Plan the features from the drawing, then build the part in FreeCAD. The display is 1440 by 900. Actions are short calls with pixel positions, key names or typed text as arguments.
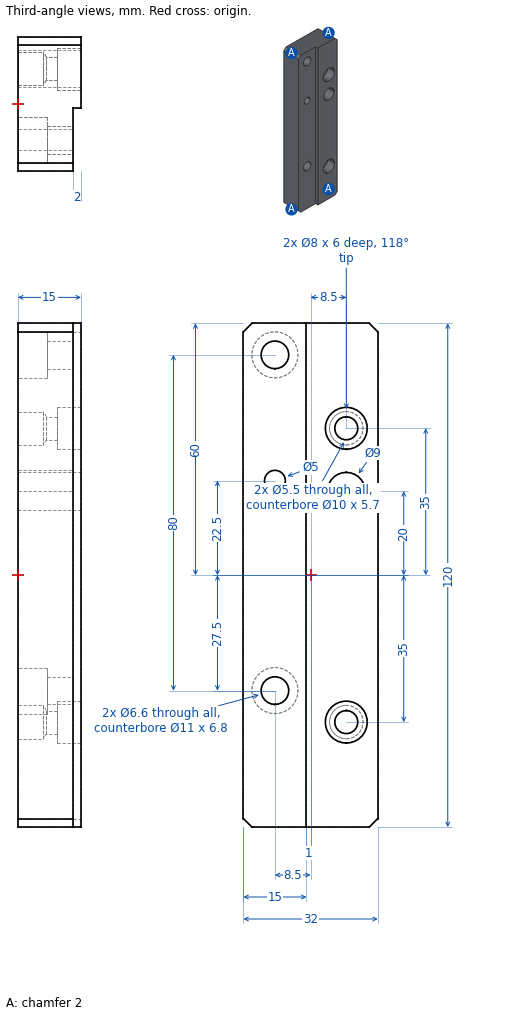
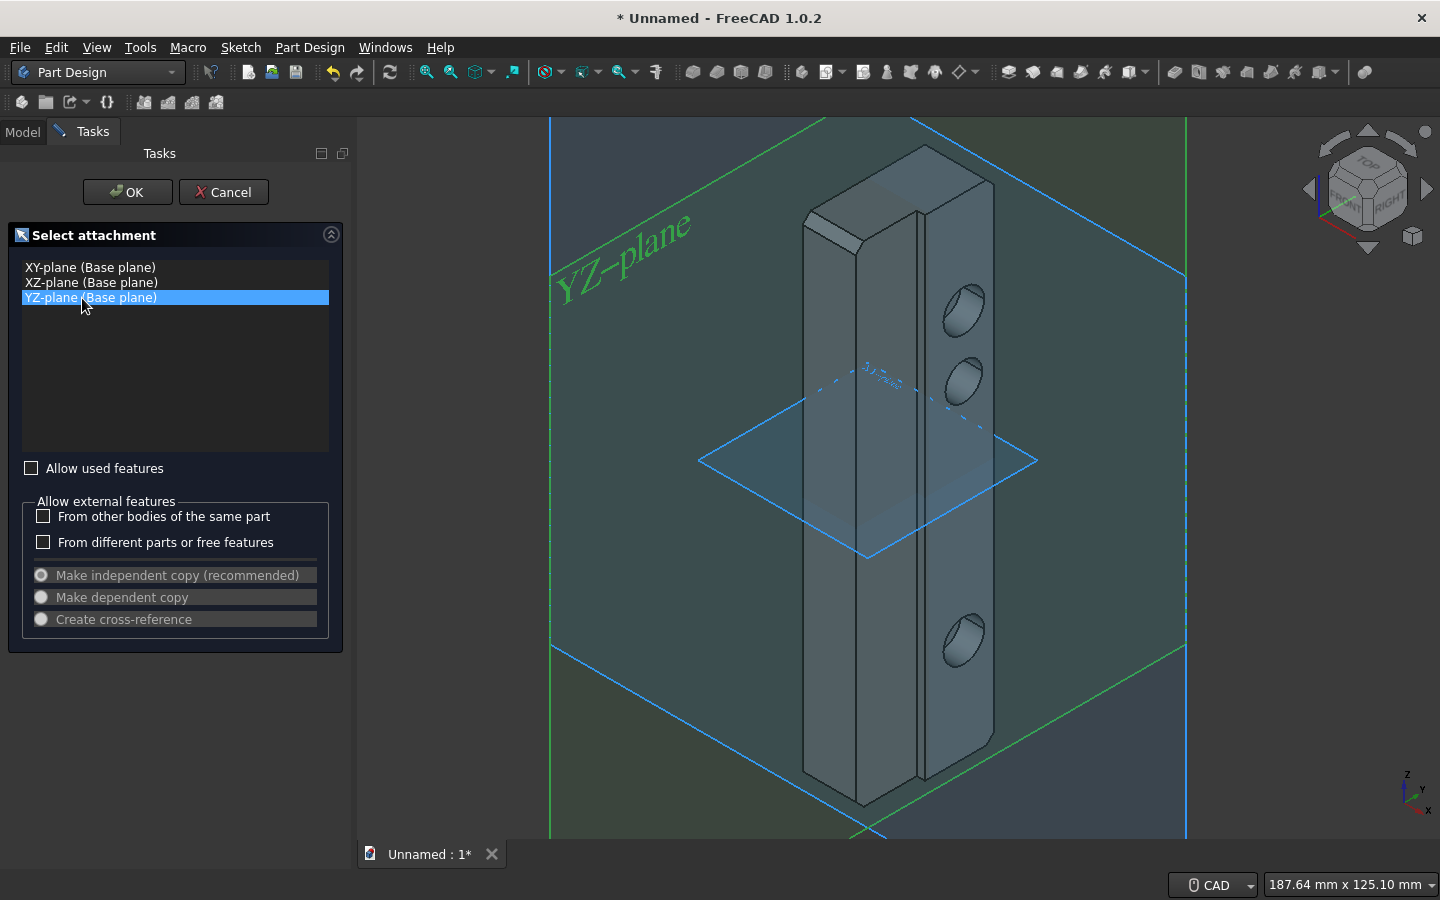
click(128, 192)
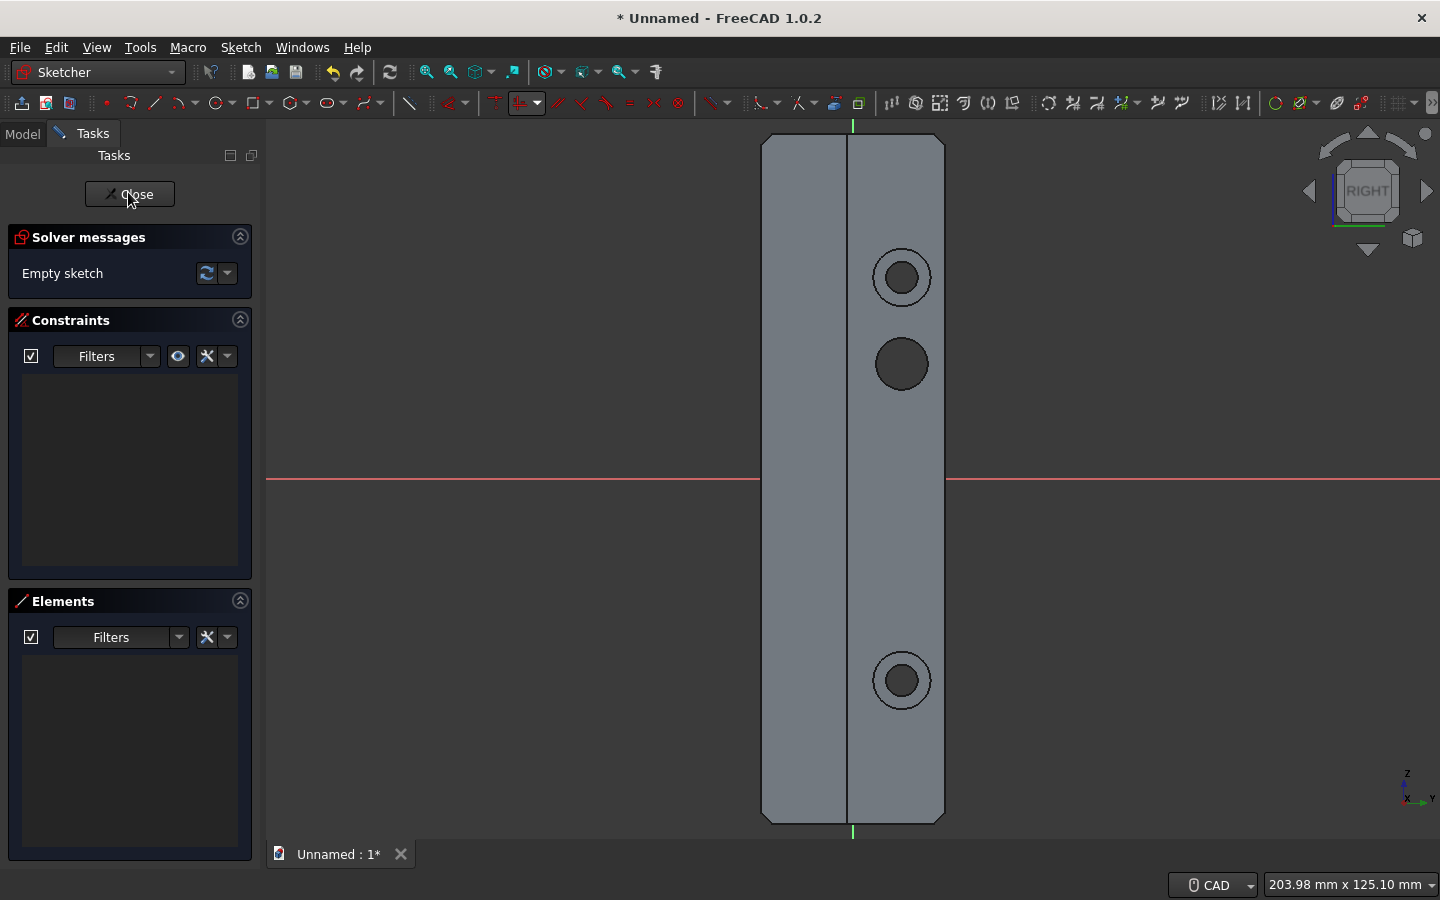
click(70, 104)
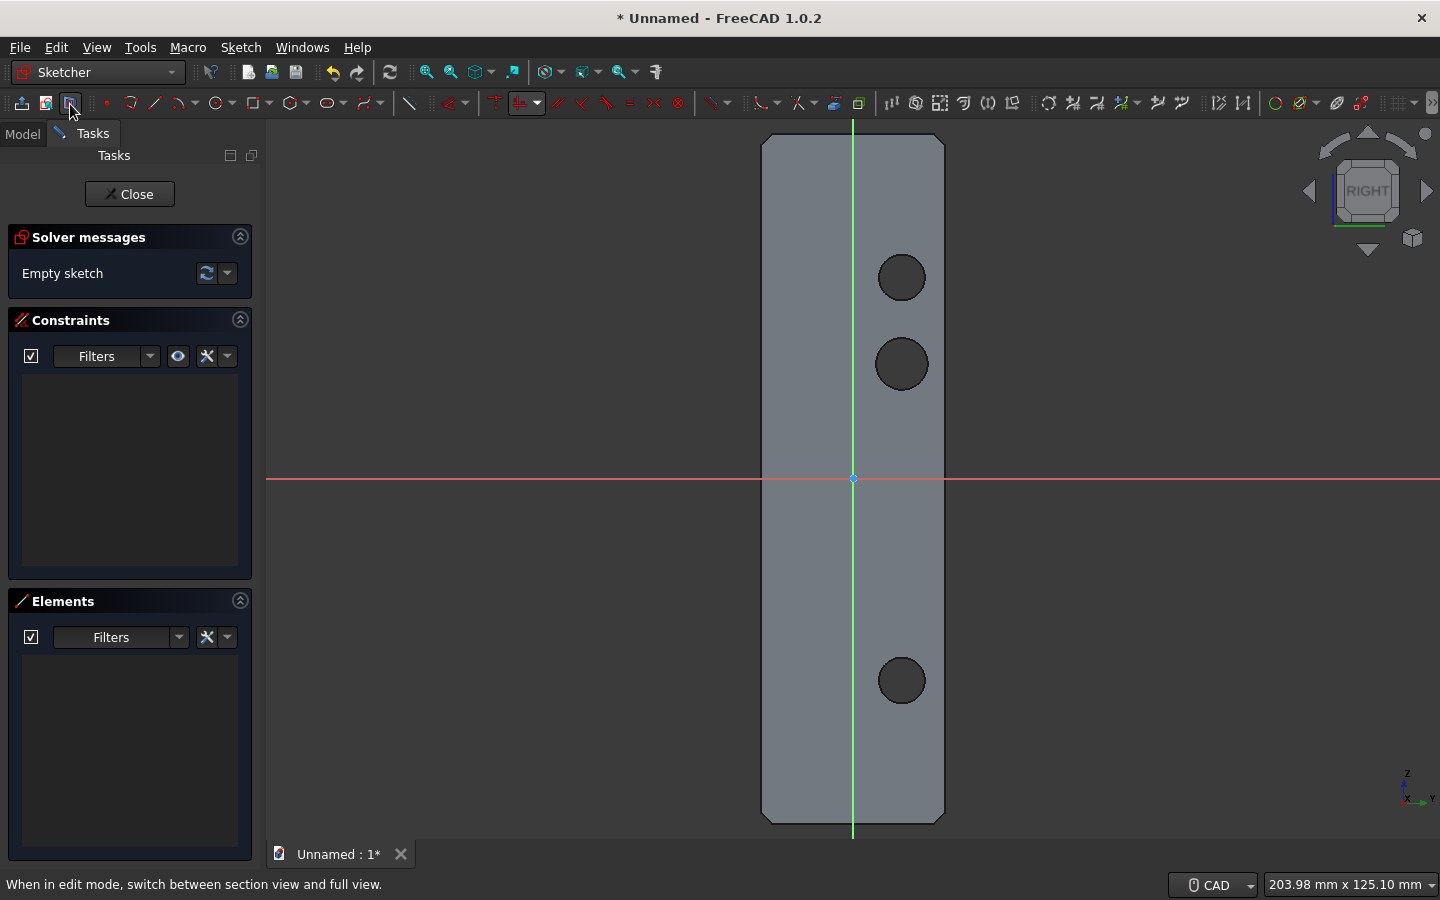
scroll(628, 804, down, 1)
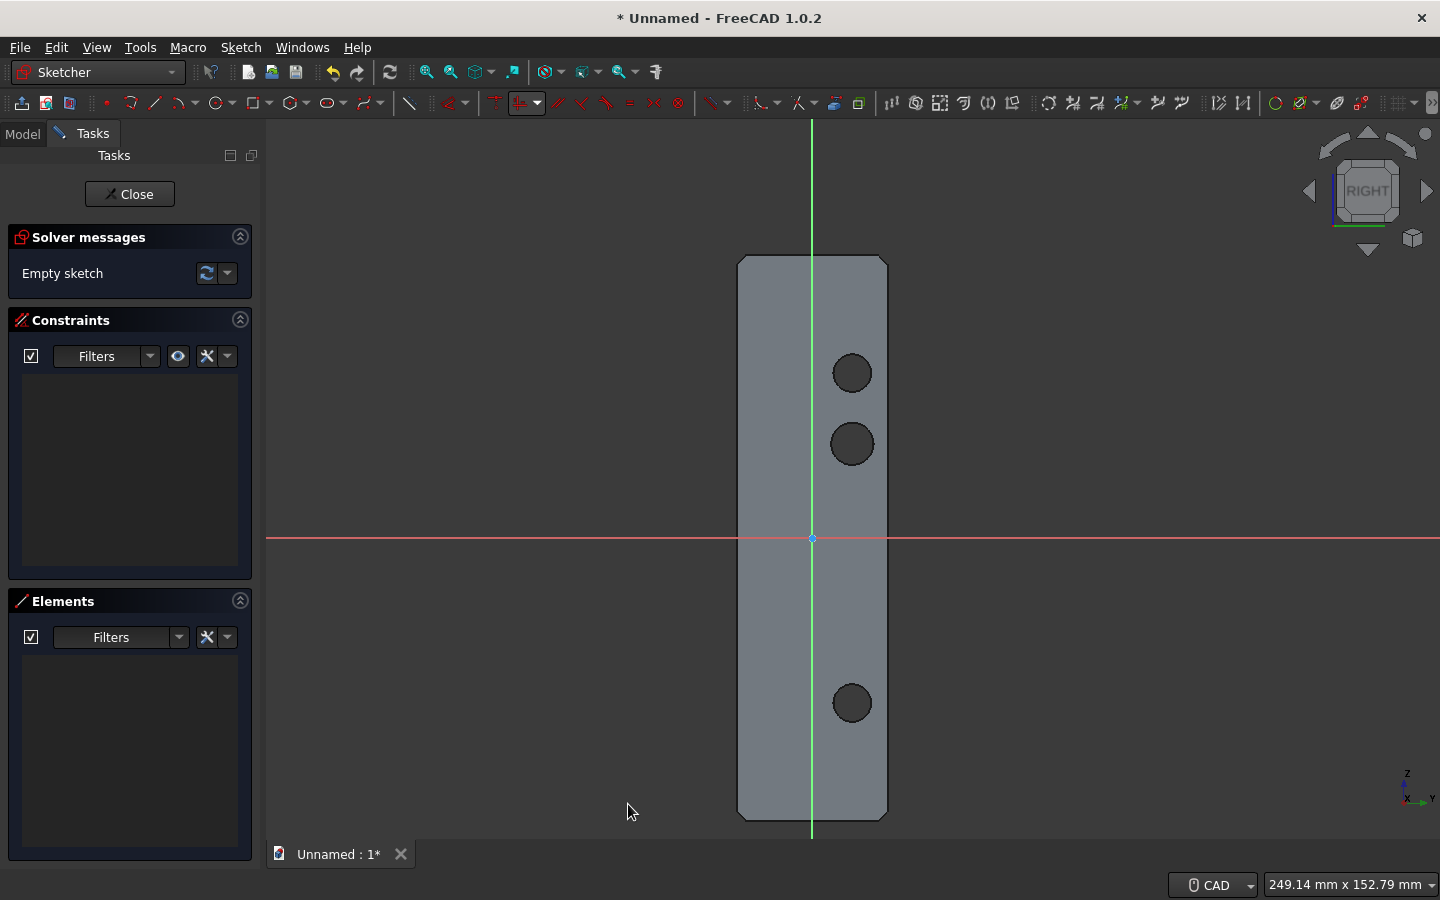
click(216, 104)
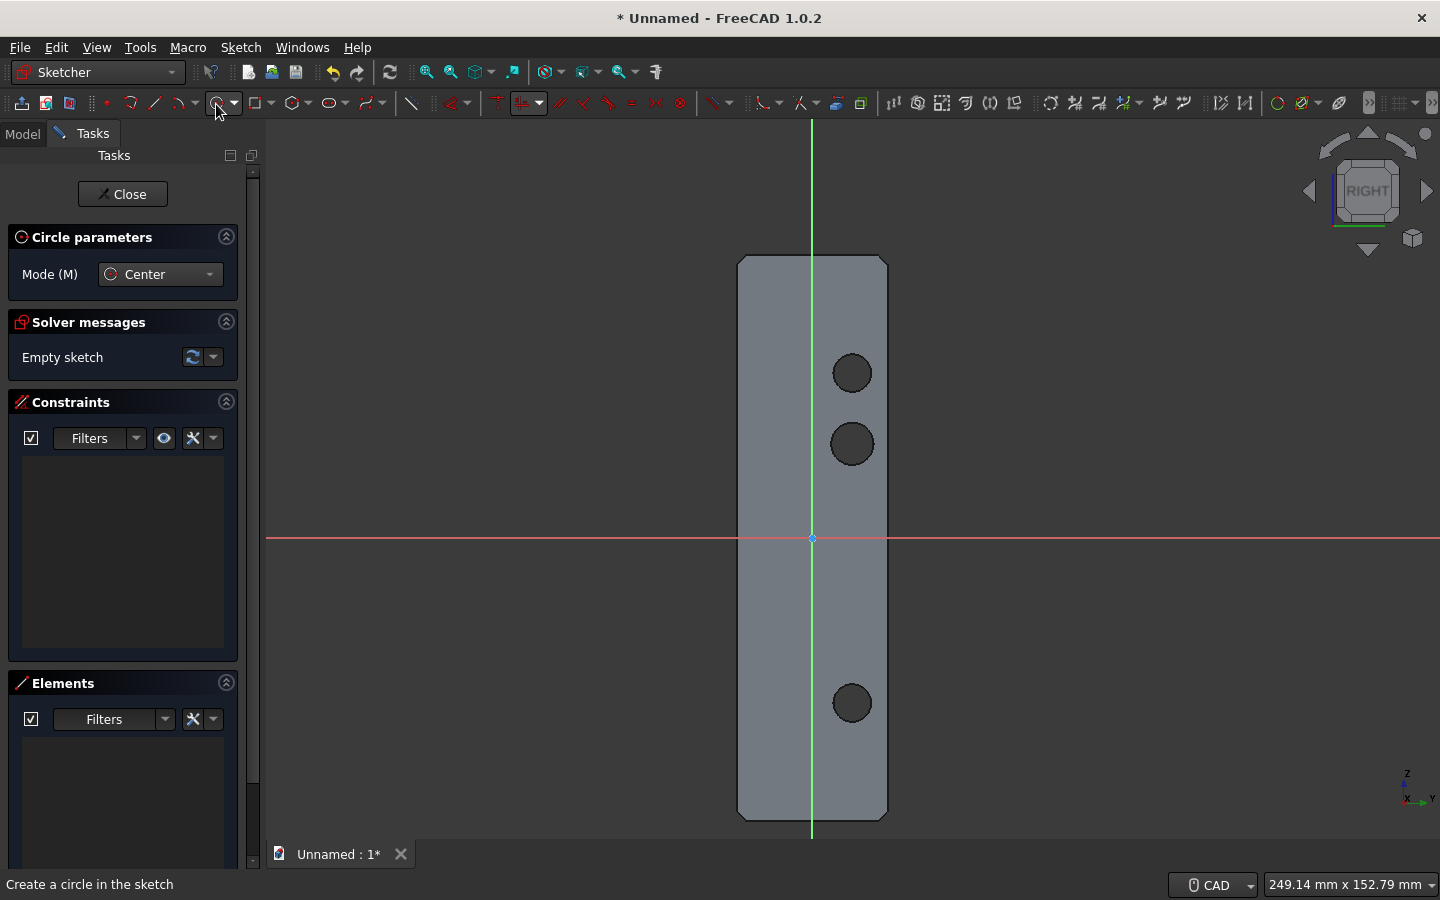
scroll(772, 668, up, 2)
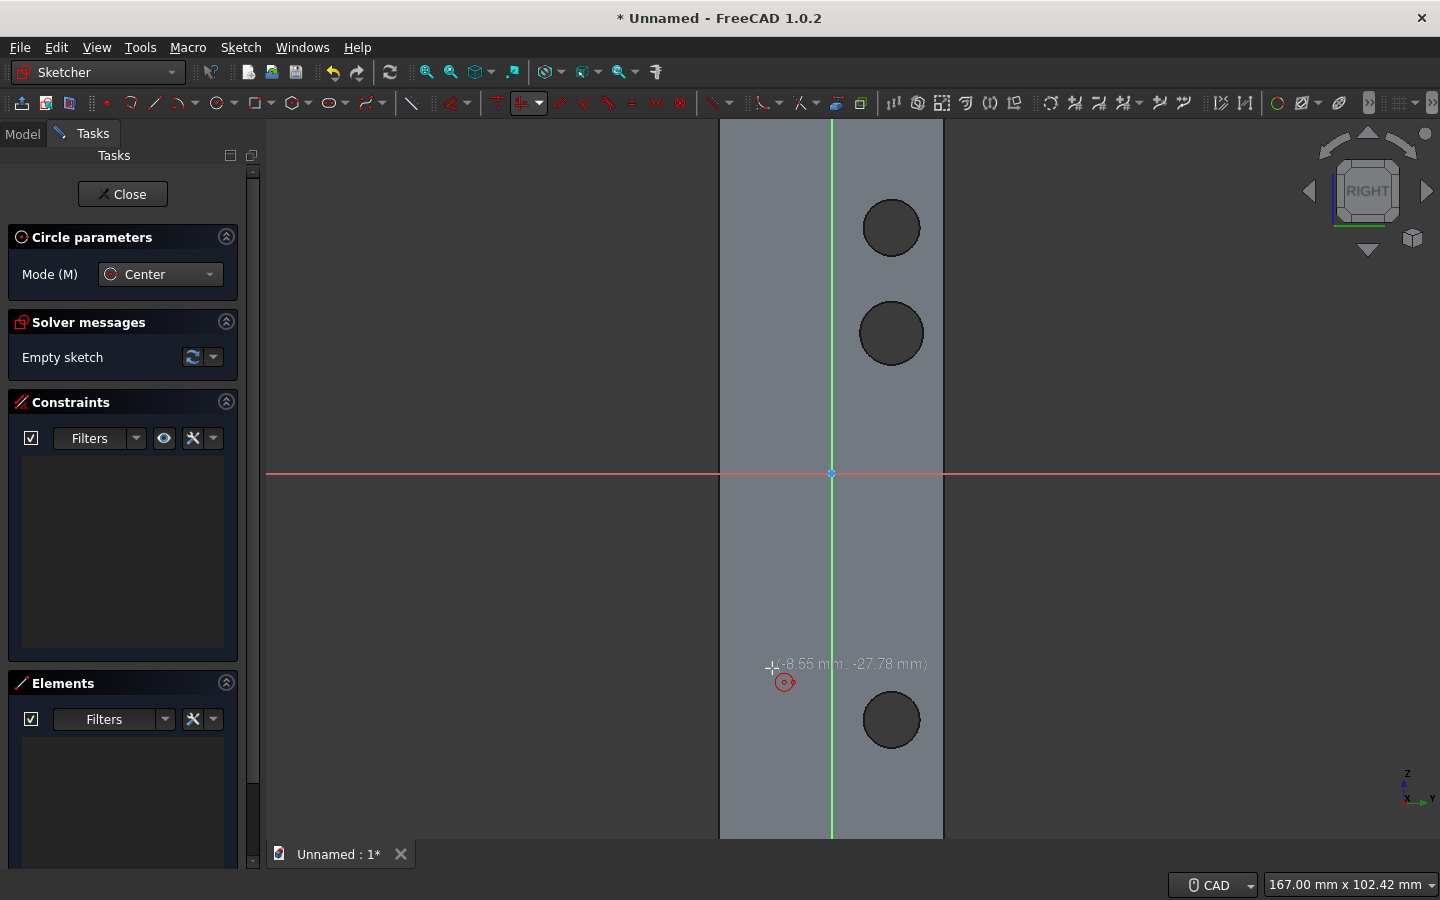
click(772, 667)
click(789, 651)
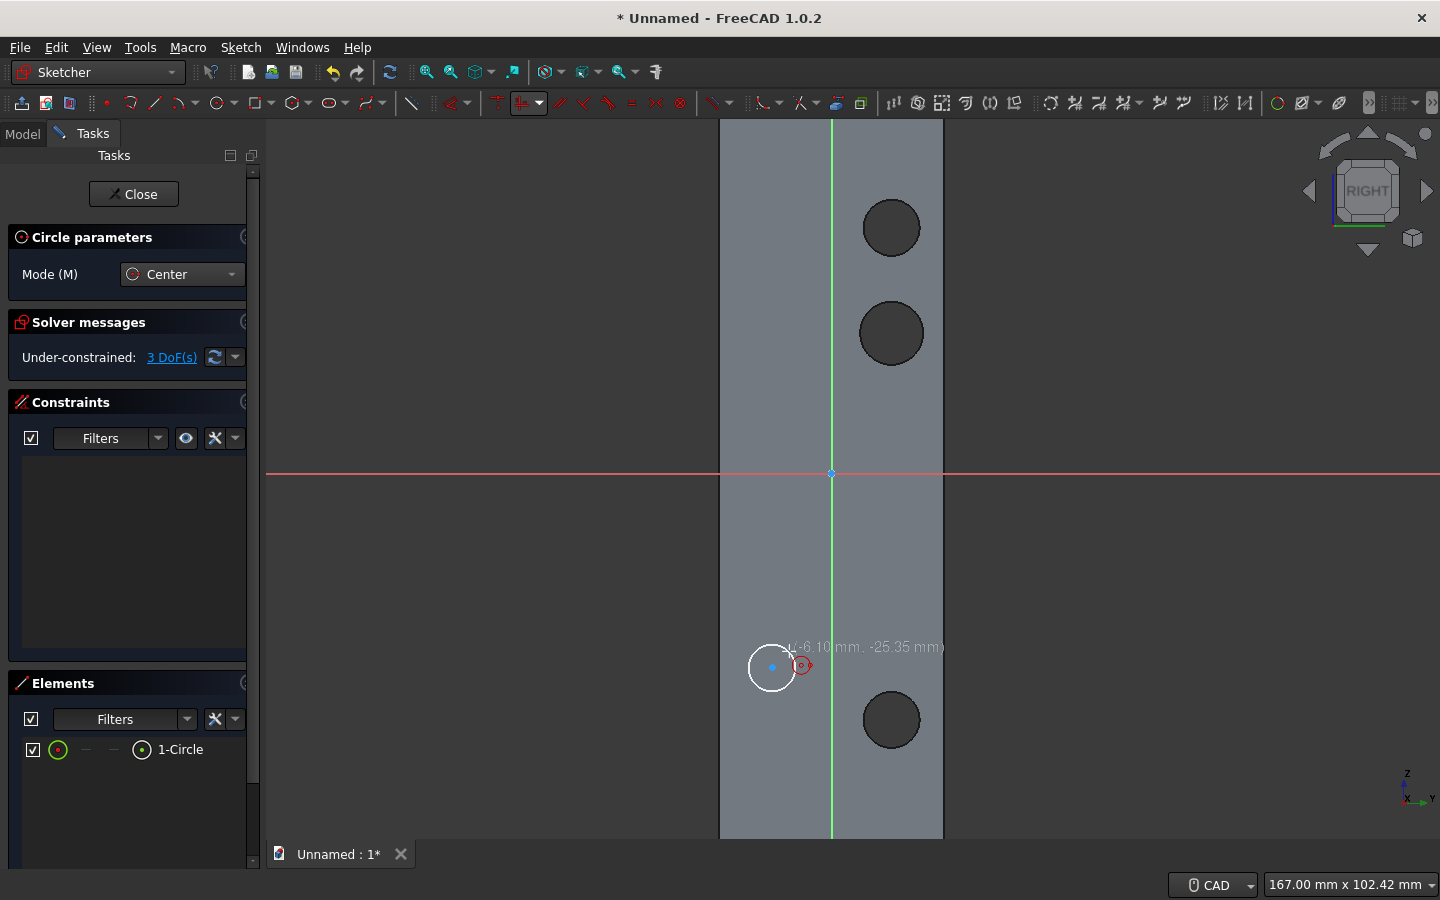
scroll(758, 811, down, 1)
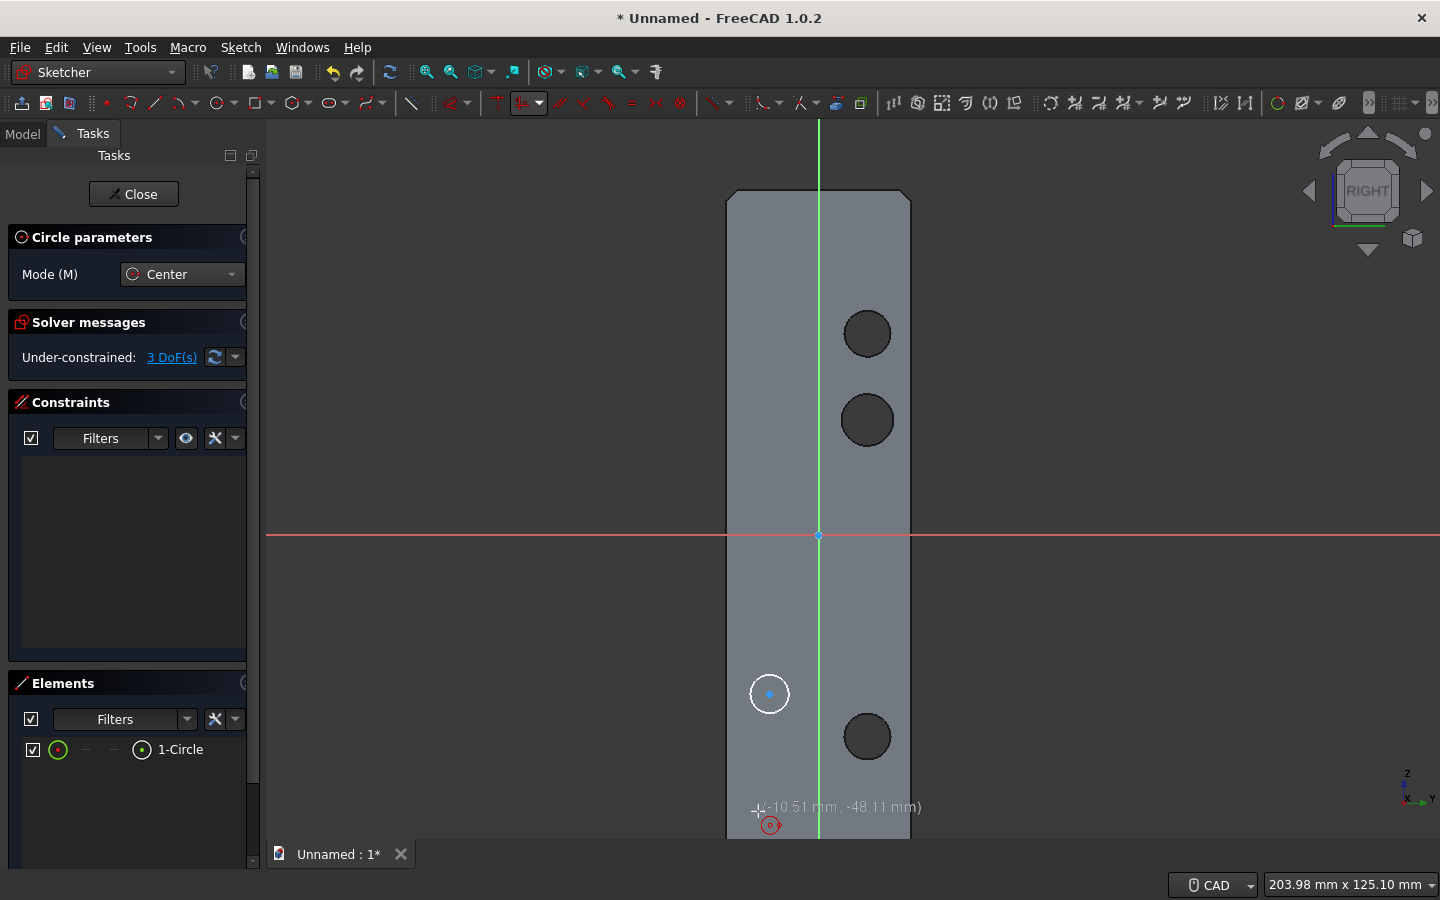
click(770, 233)
click(783, 220)
key(Escape)